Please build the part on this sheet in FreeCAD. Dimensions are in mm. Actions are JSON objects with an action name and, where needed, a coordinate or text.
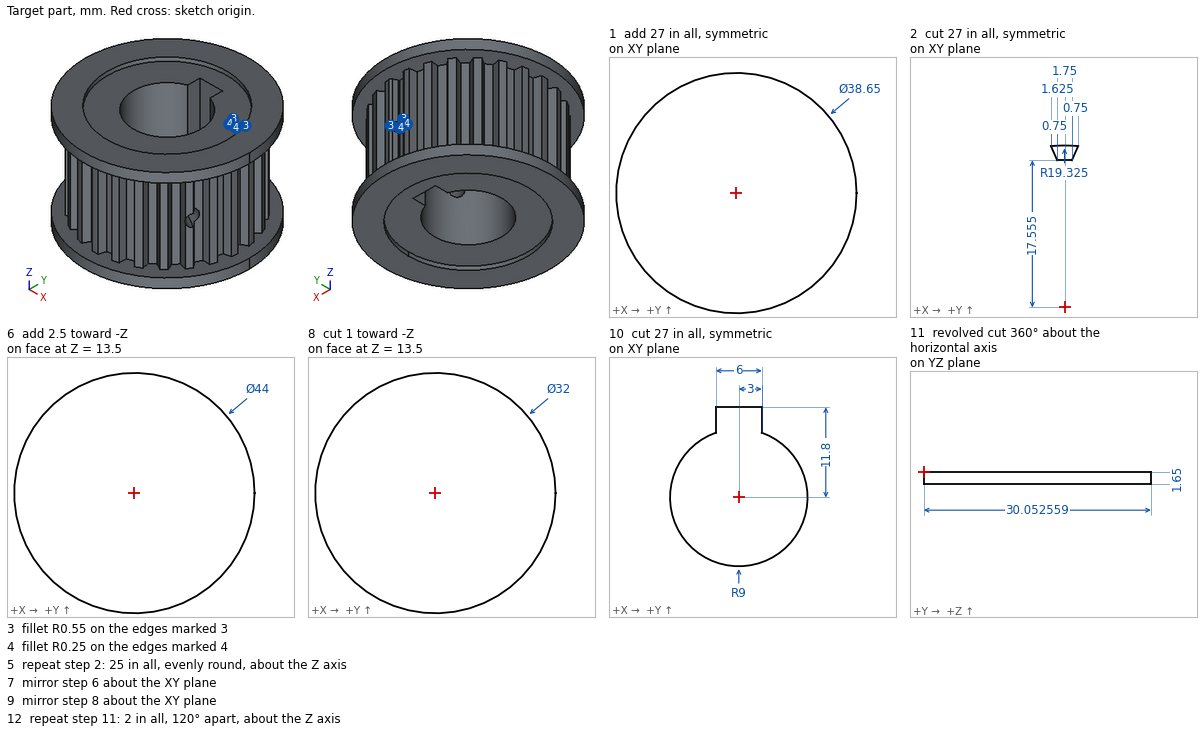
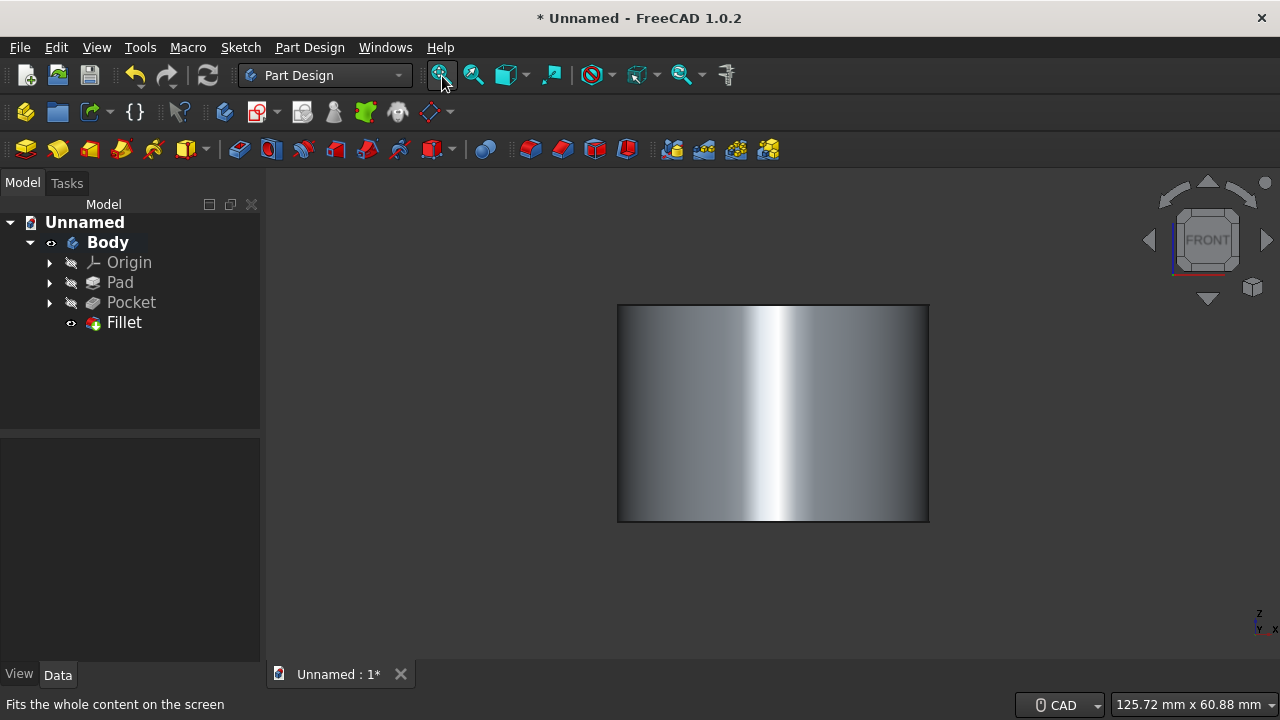
{"action": "key", "text": "3"}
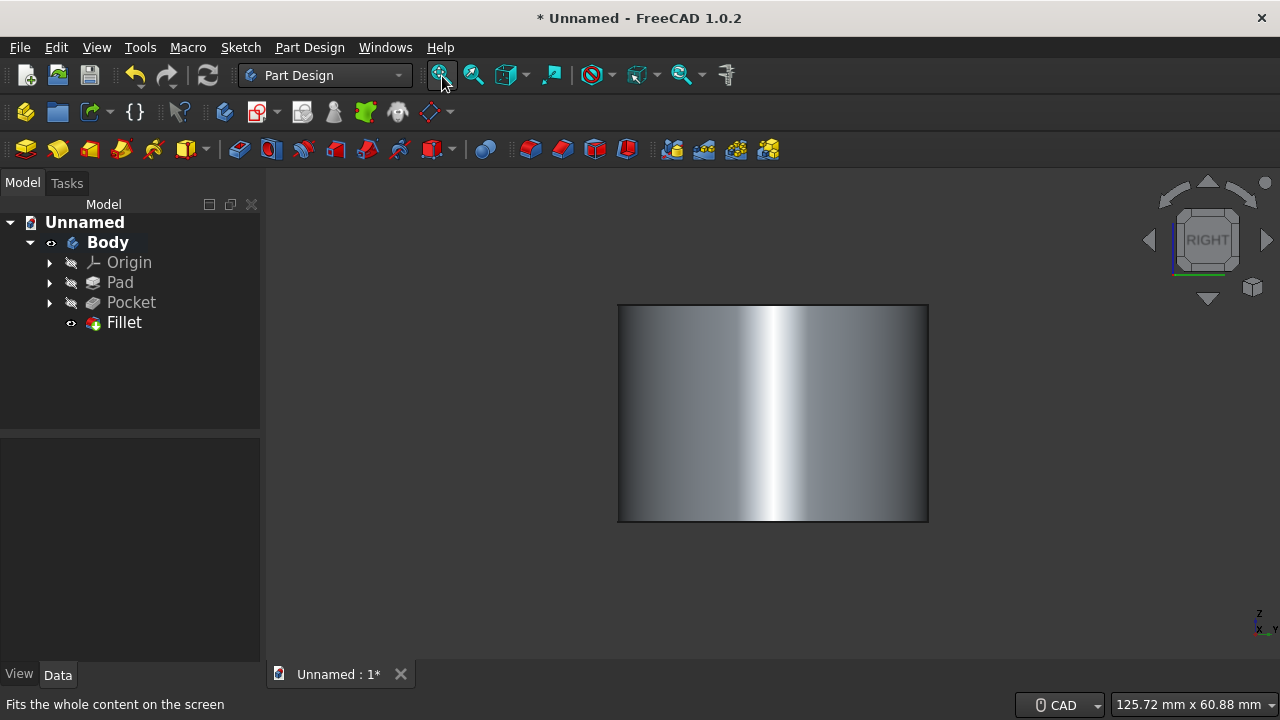
{"action": "left_click", "coordinate": [442, 76]}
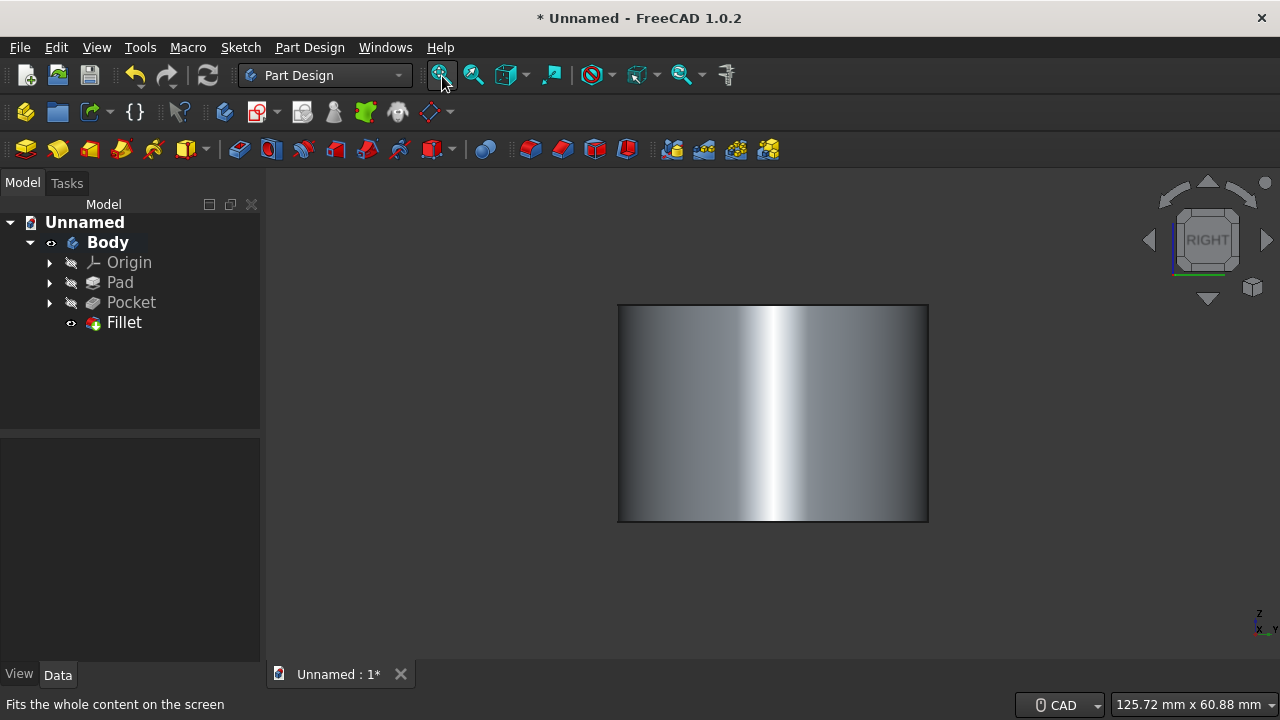
{"action": "key", "text": "5"}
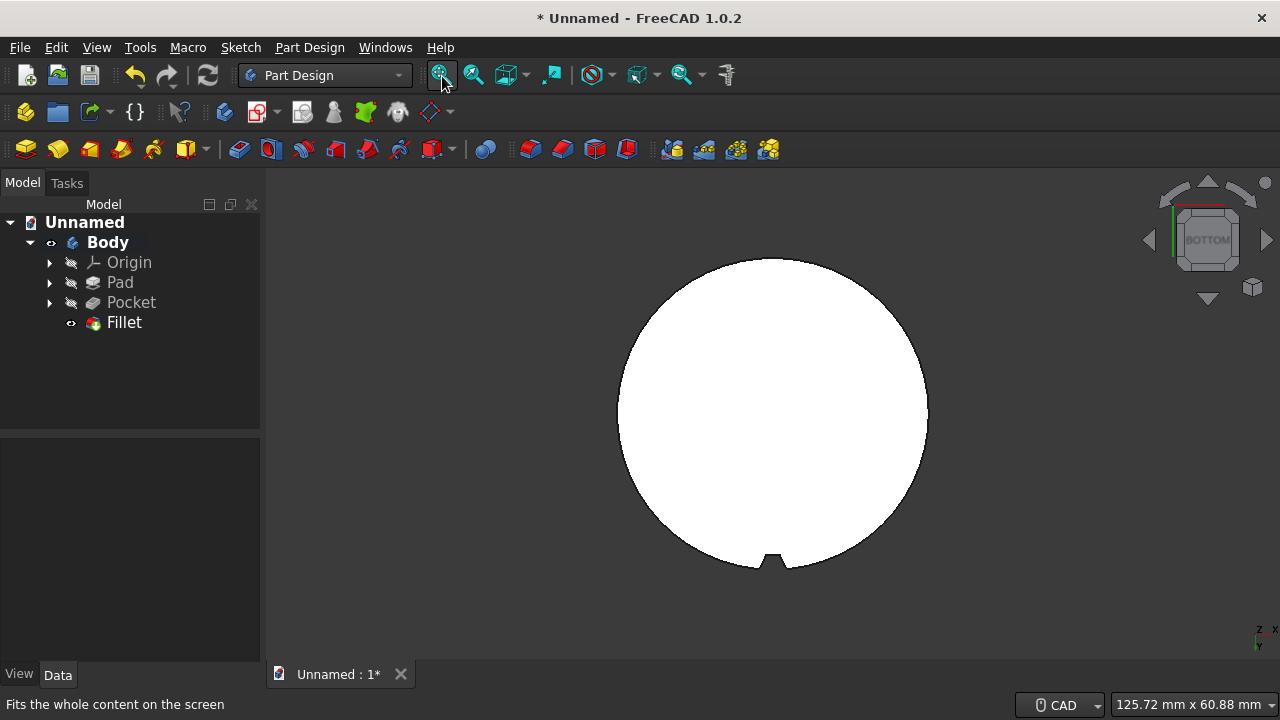
{"action": "key", "text": "4"}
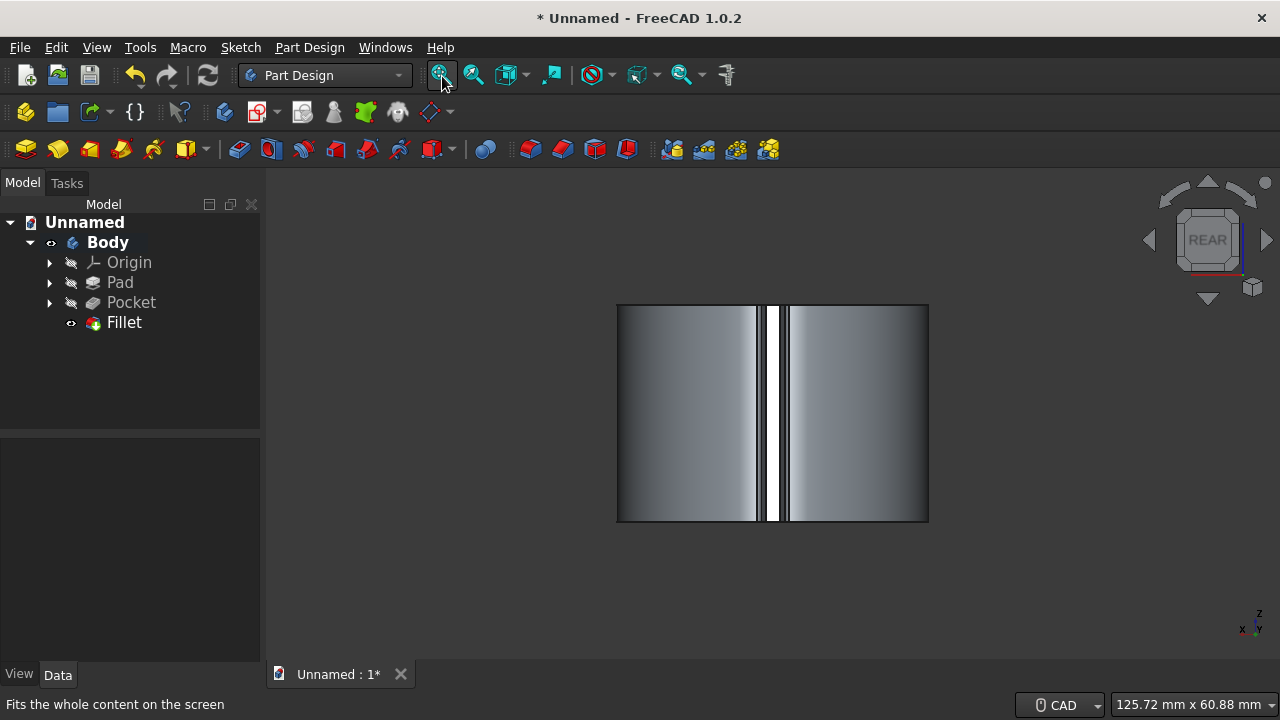
{"action": "left_click", "coordinate": [442, 76]}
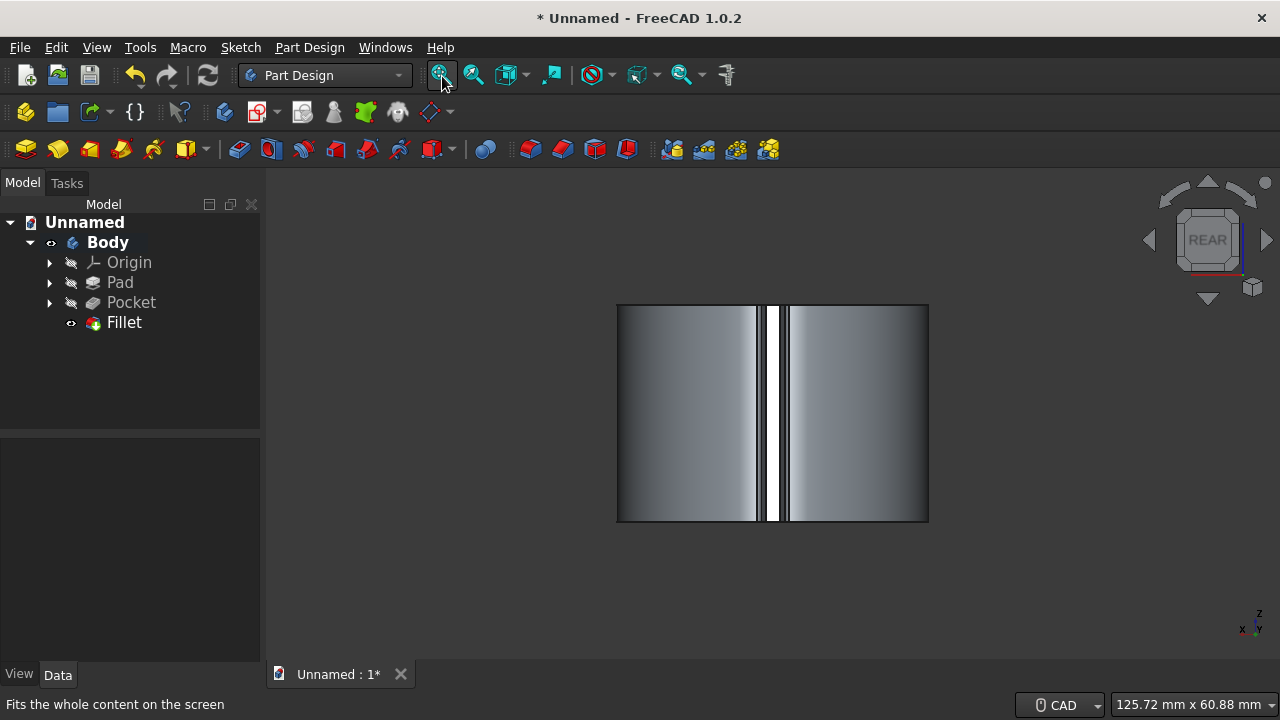
{"action": "key", "text": "6"}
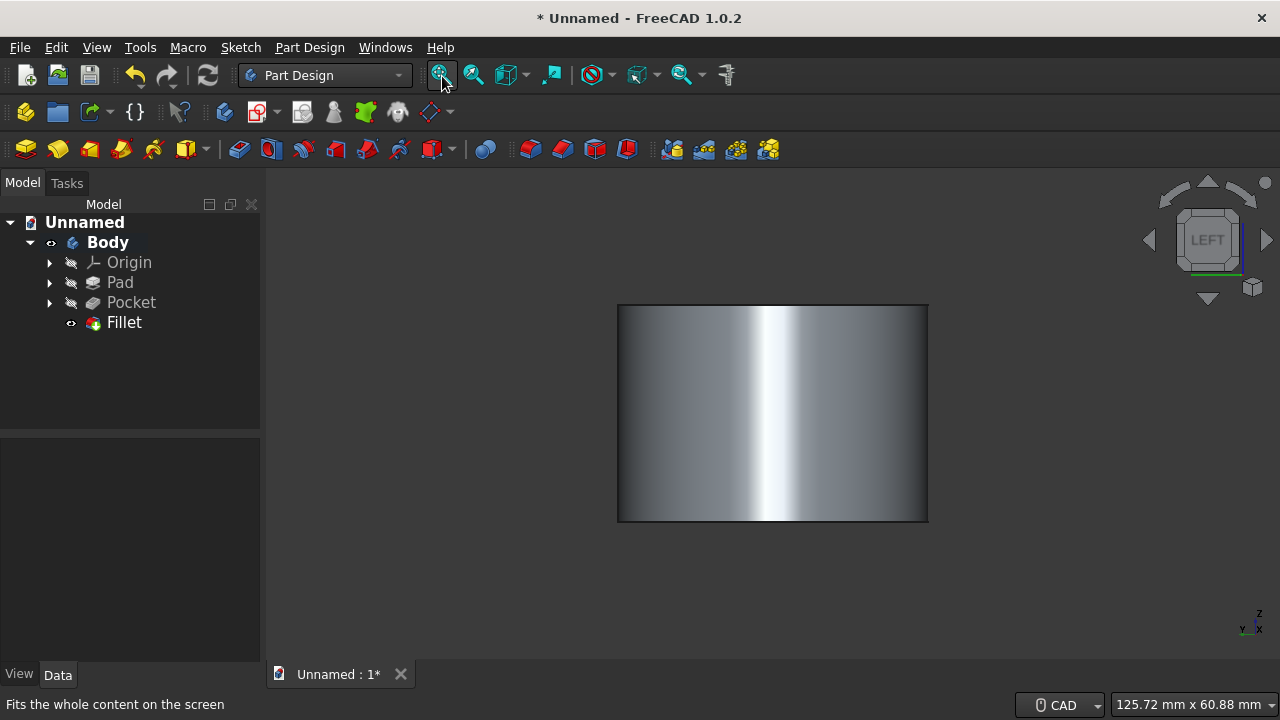
{"action": "left_click", "coordinate": [442, 76]}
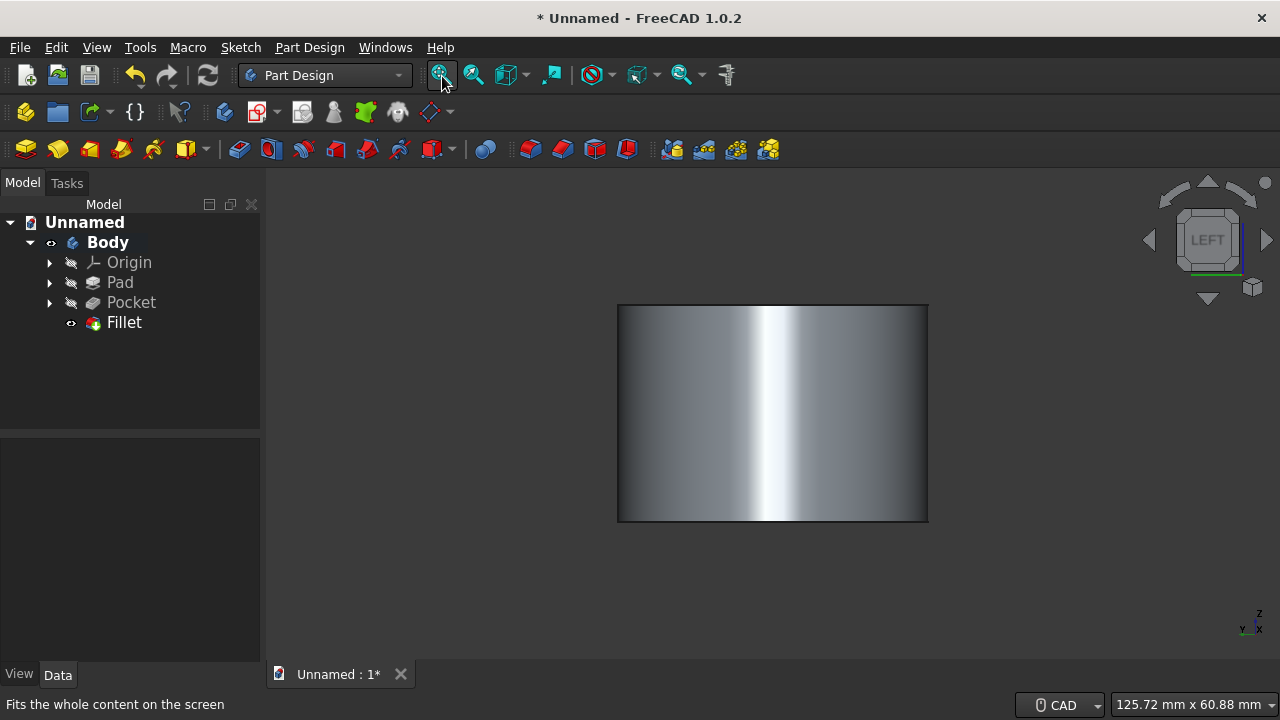
{"action": "key", "text": "v 3"}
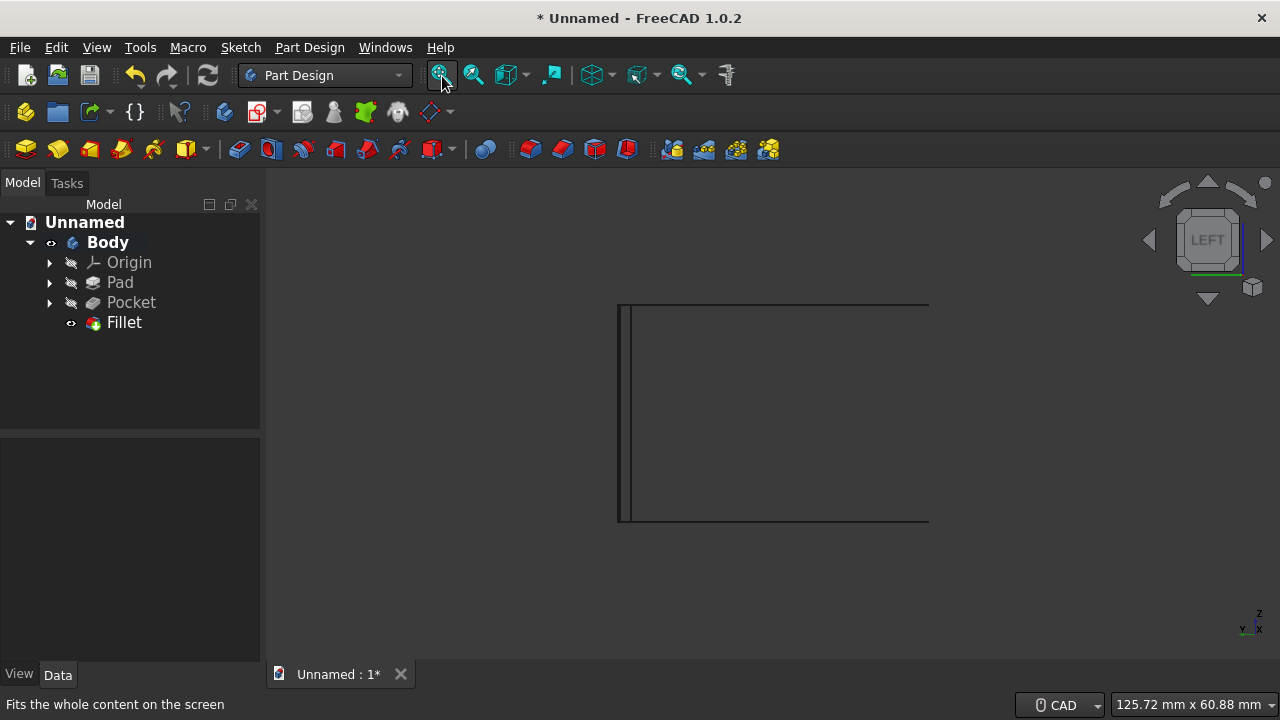
{"action": "key", "text": "0"}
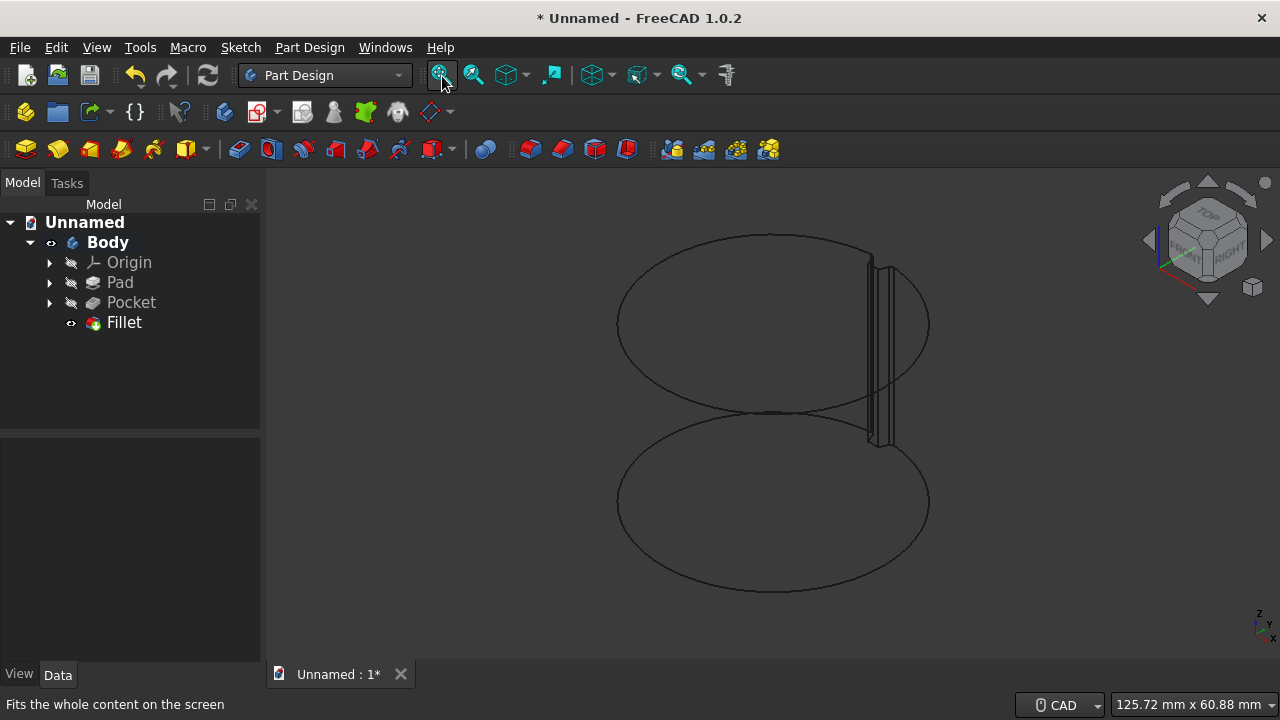
{"action": "left_click", "coordinate": [868, 352]}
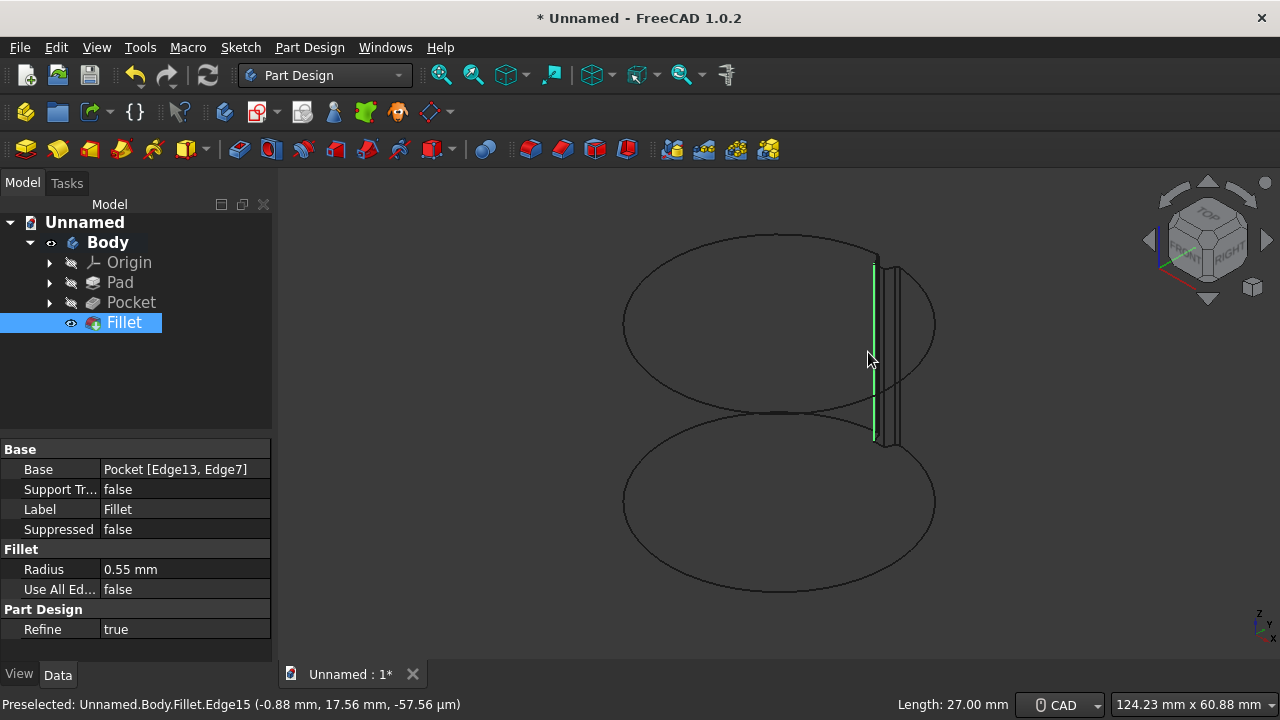
{"action": "left_click", "coordinate": [884, 357], "text": "ctrl"}